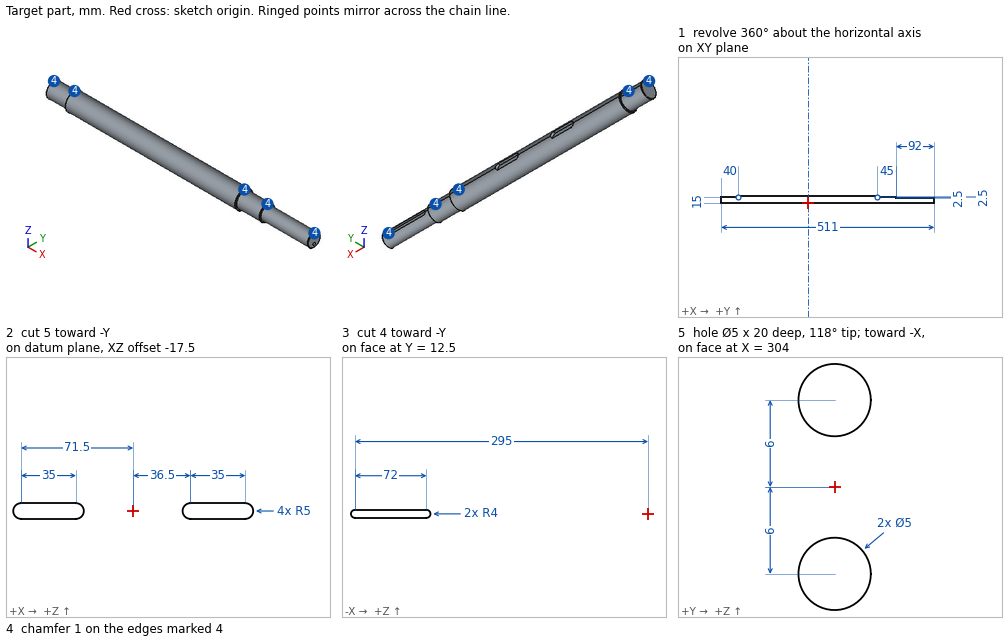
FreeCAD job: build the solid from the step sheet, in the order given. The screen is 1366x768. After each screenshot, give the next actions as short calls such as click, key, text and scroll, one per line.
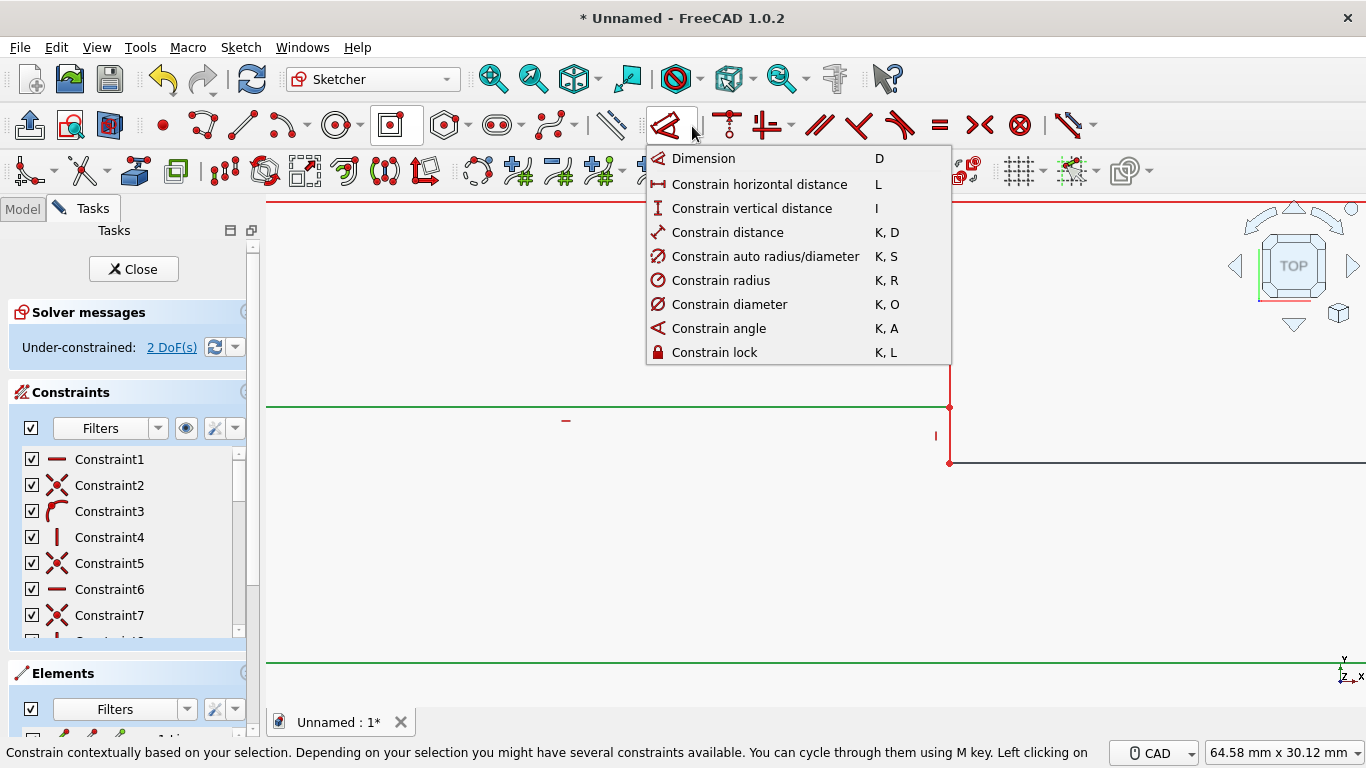
click(799, 208)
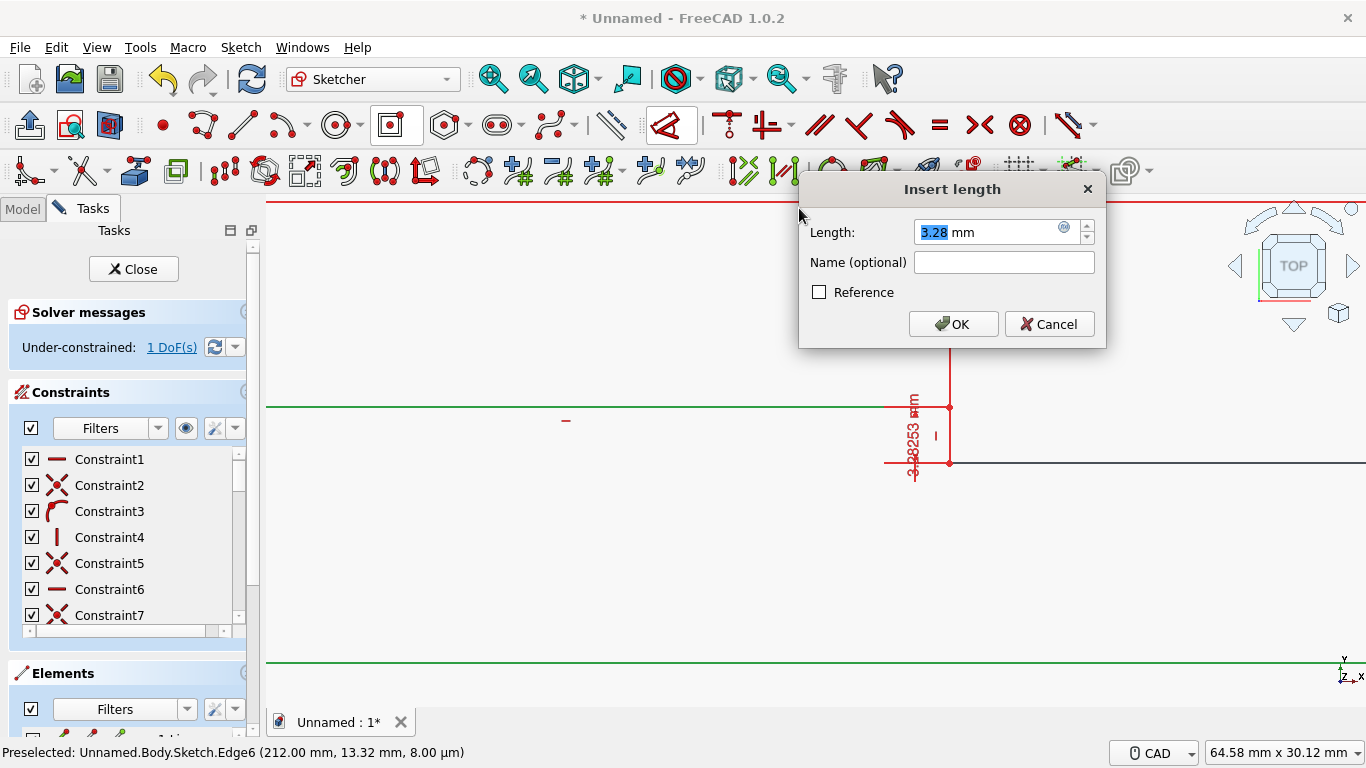
text(2.5)
key(Return)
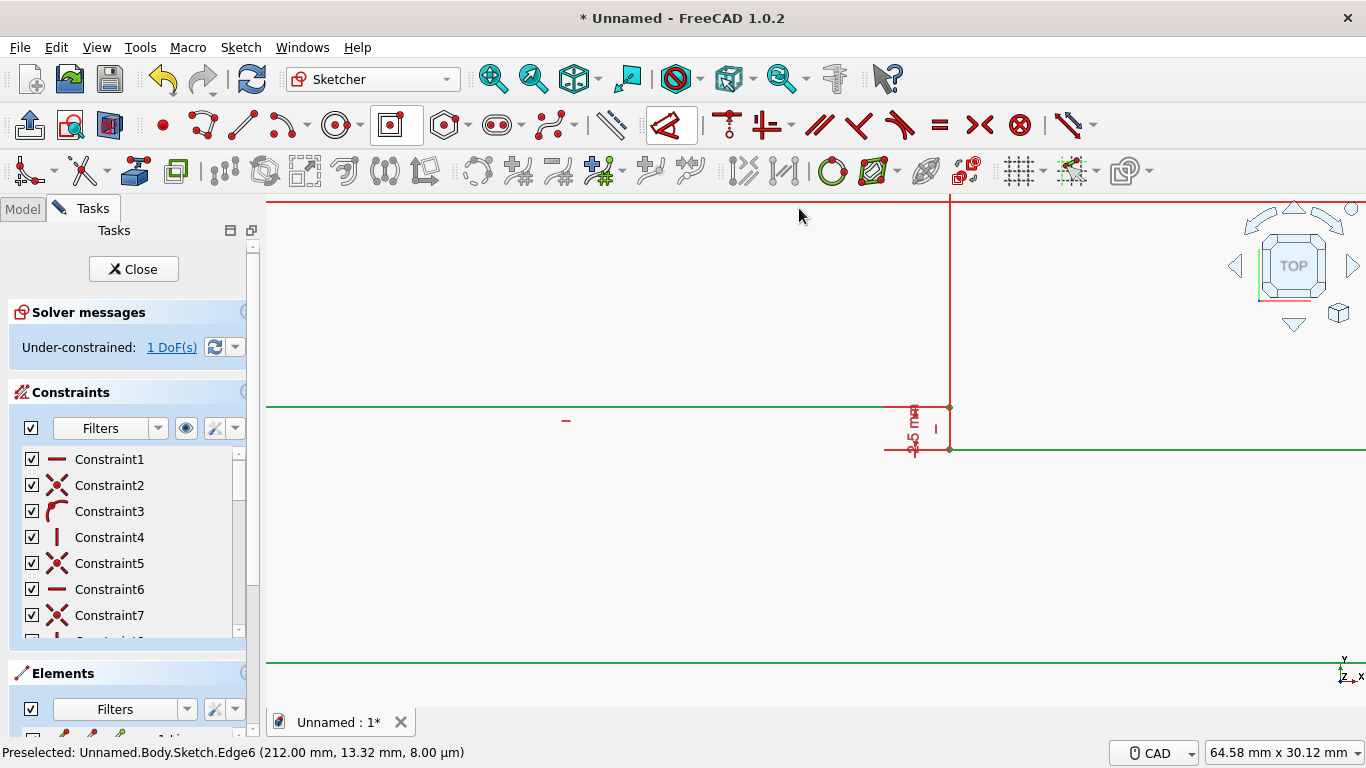
scroll(955, 445, down, 13)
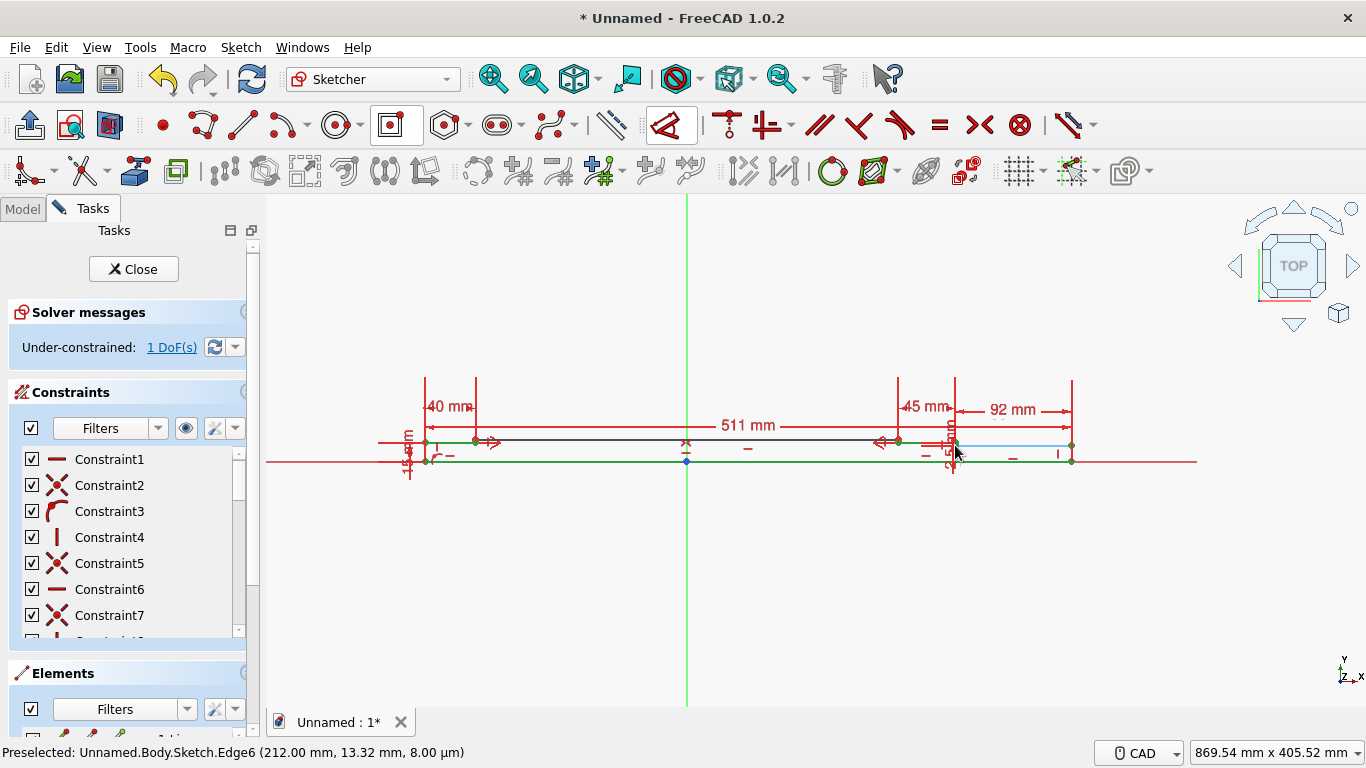
scroll(898, 442, up, 14)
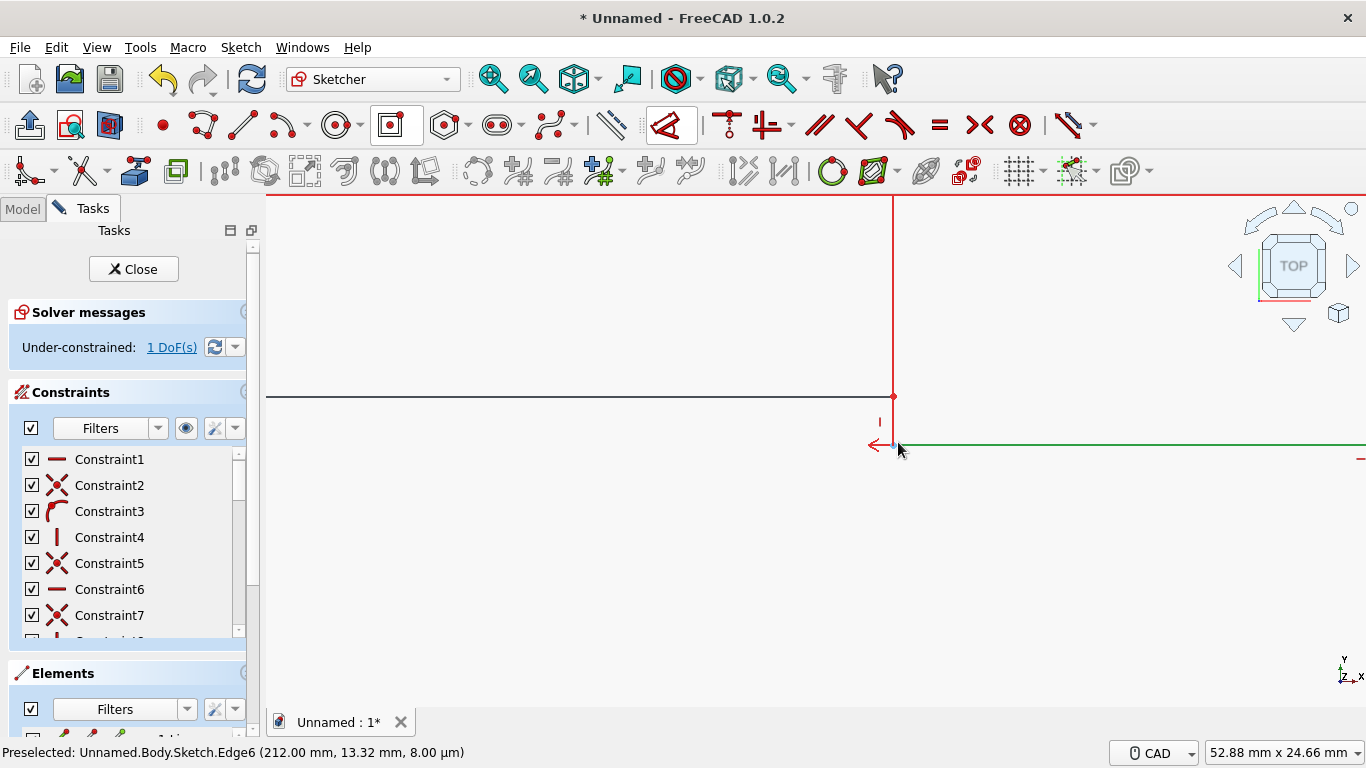
click(893, 431)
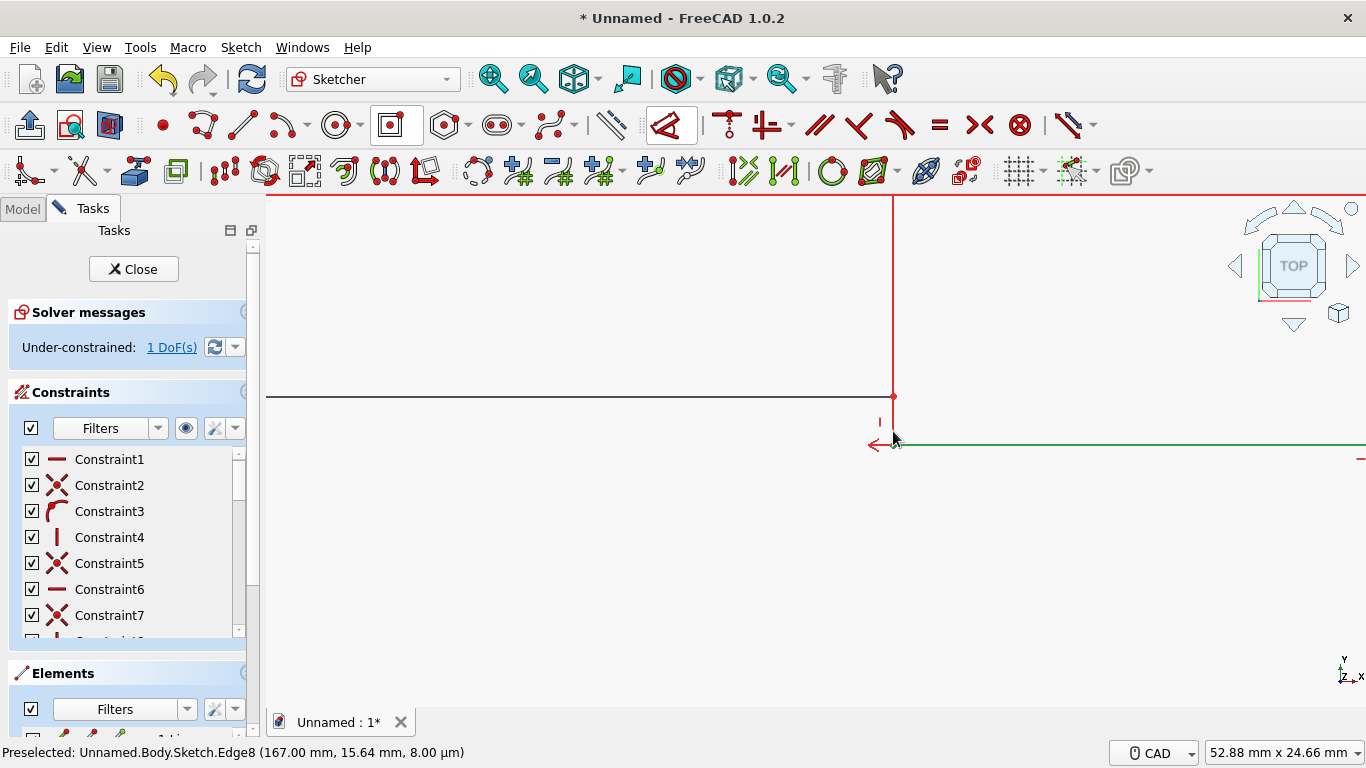
key(i)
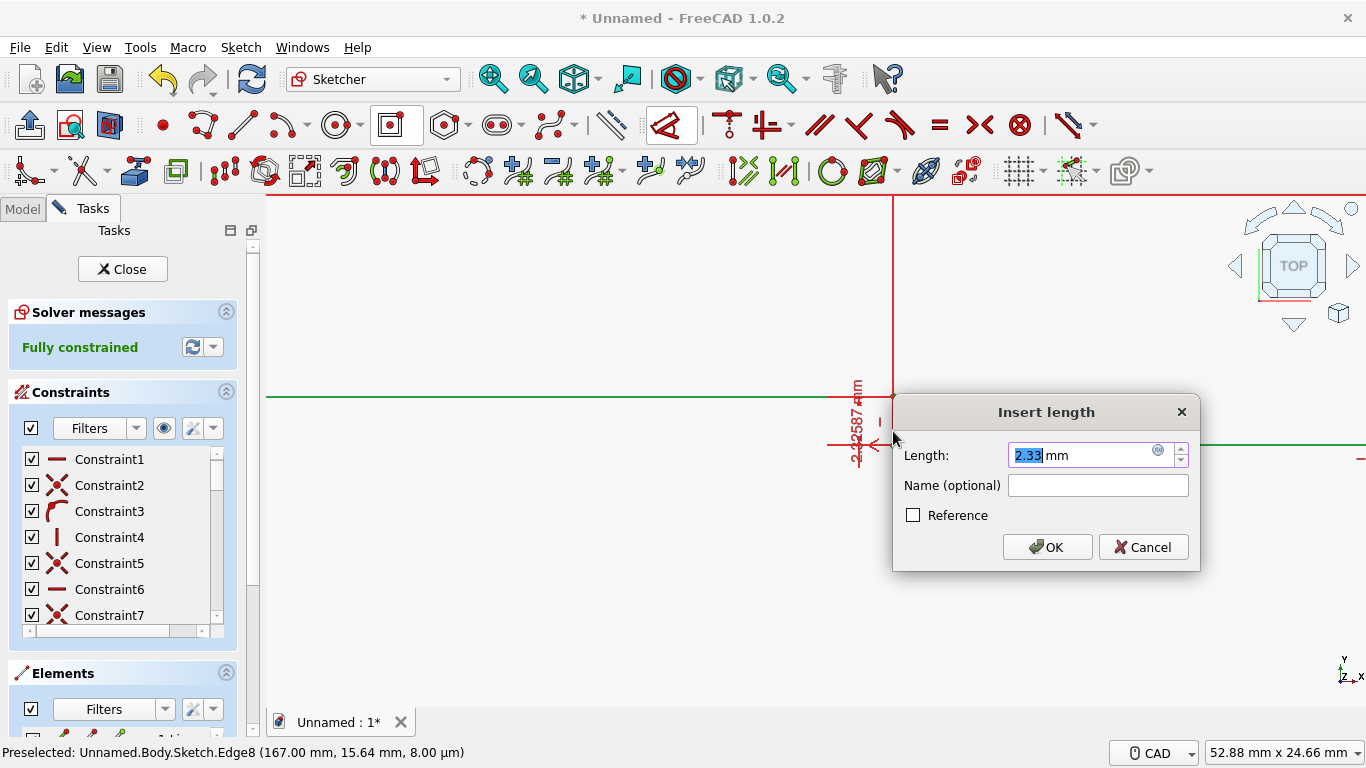
text(2.5)
key(Return)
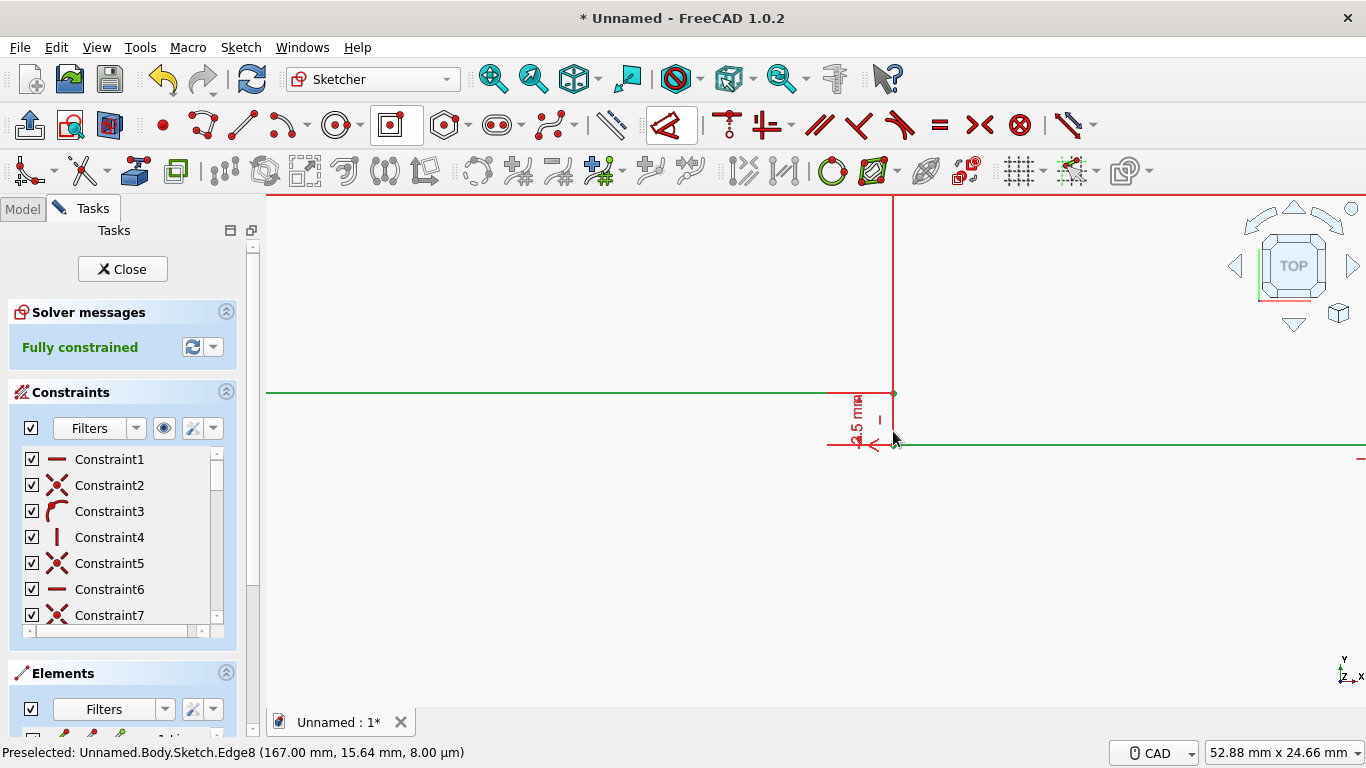
click(123, 269)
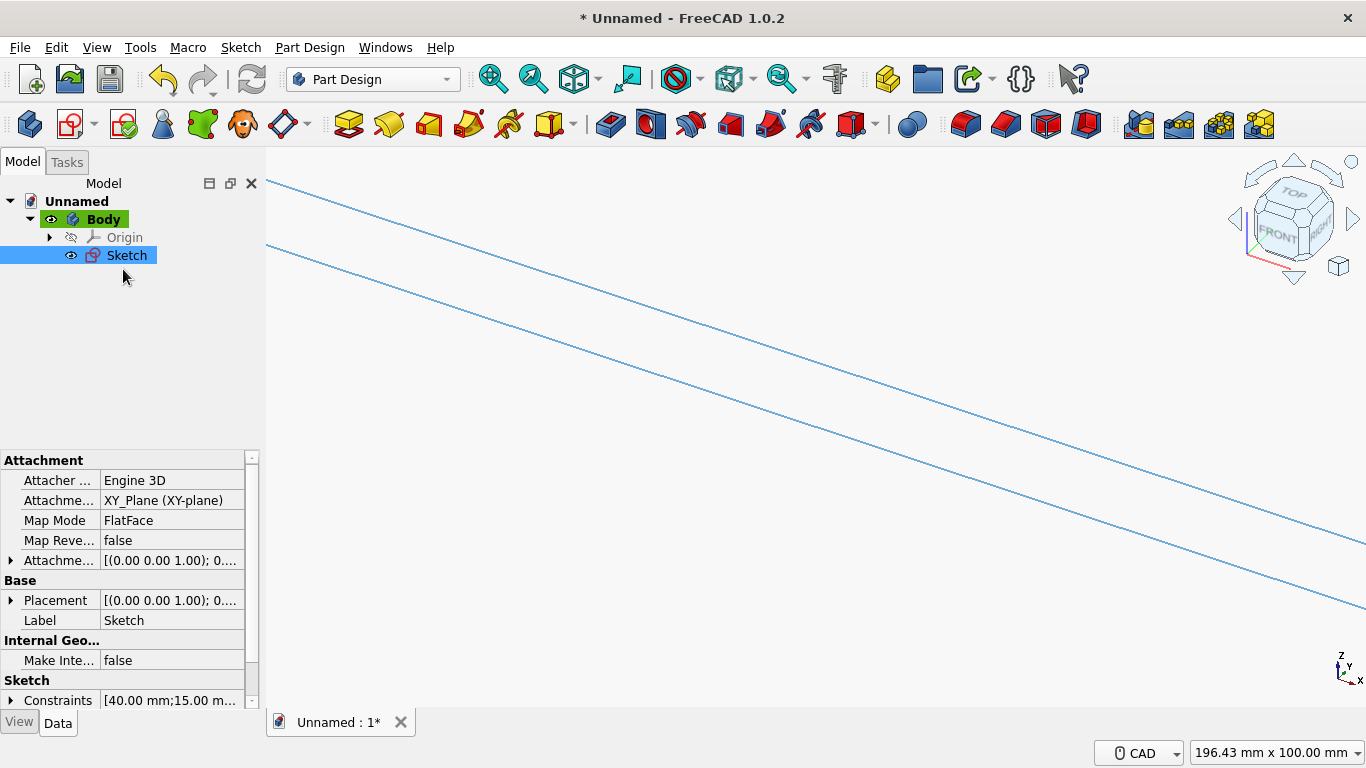
click(390, 124)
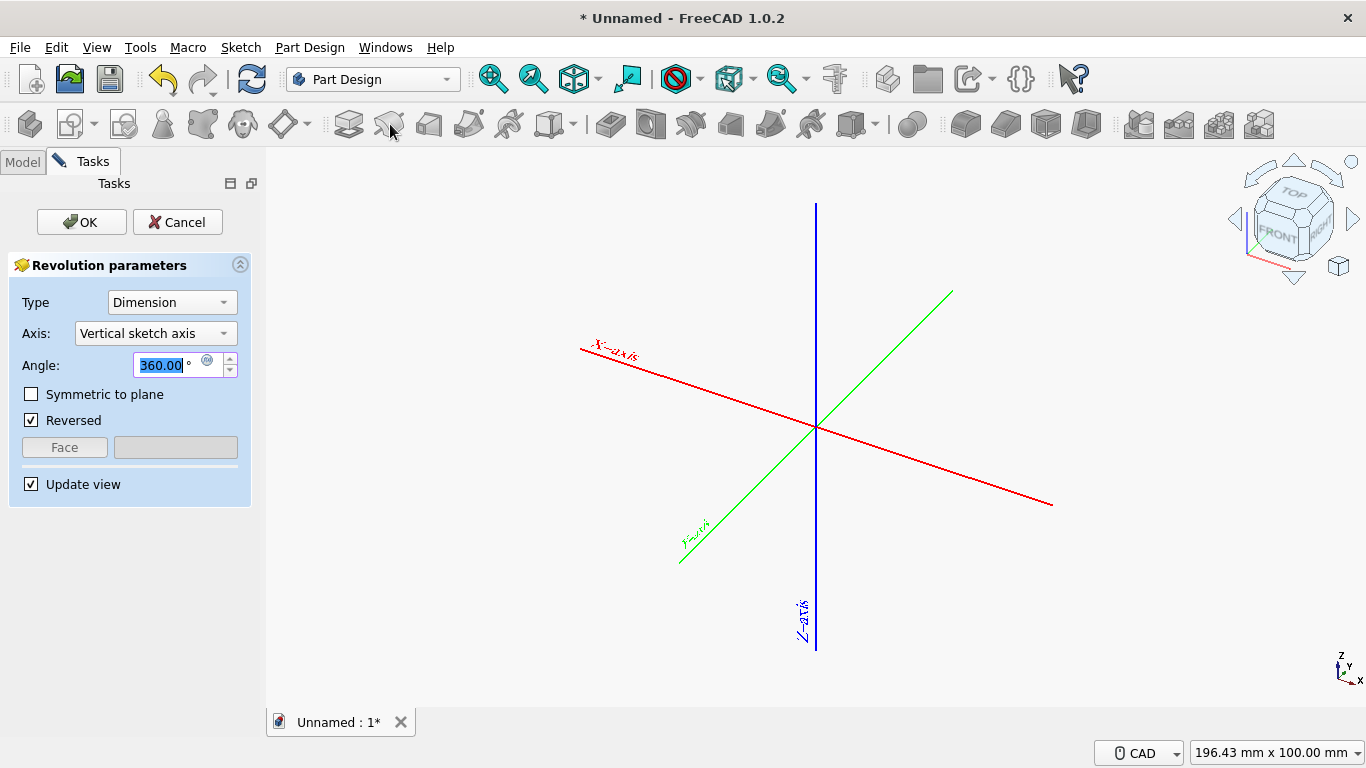
click(156, 334)